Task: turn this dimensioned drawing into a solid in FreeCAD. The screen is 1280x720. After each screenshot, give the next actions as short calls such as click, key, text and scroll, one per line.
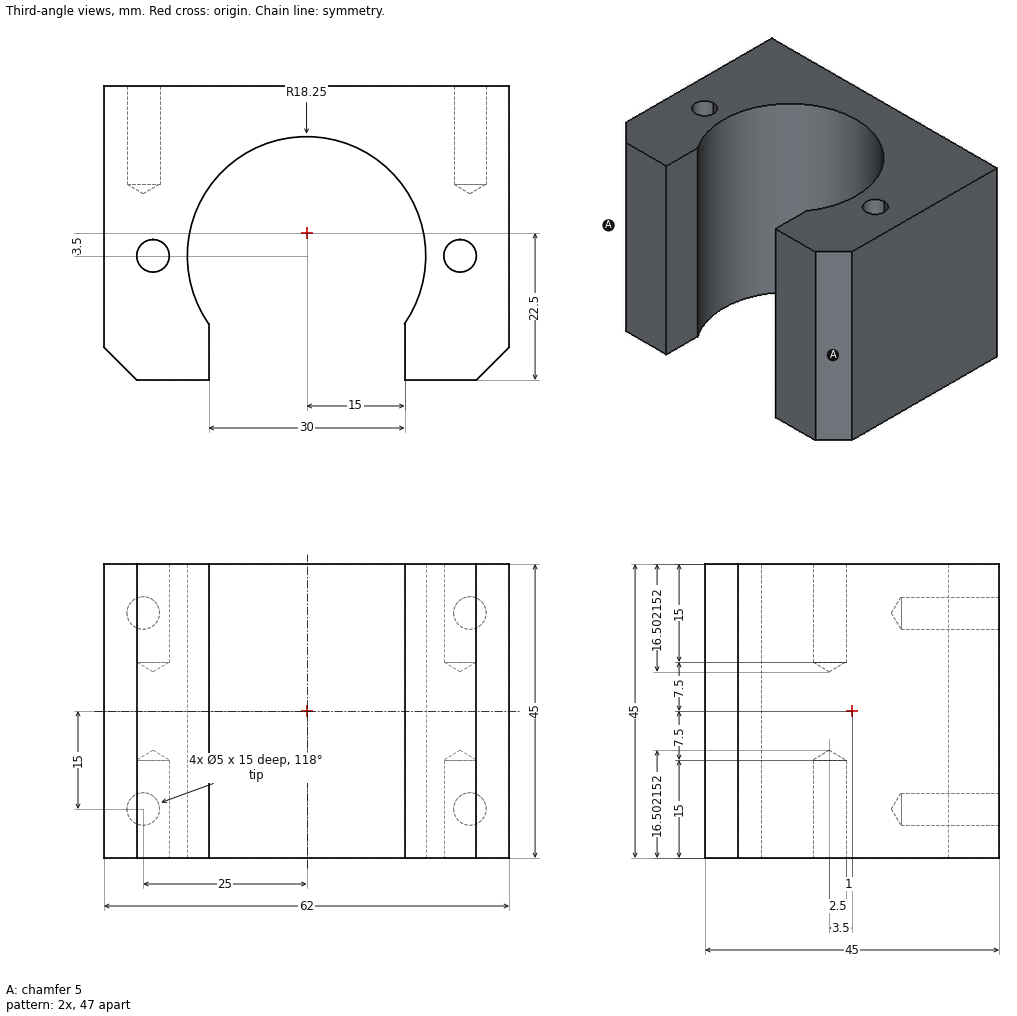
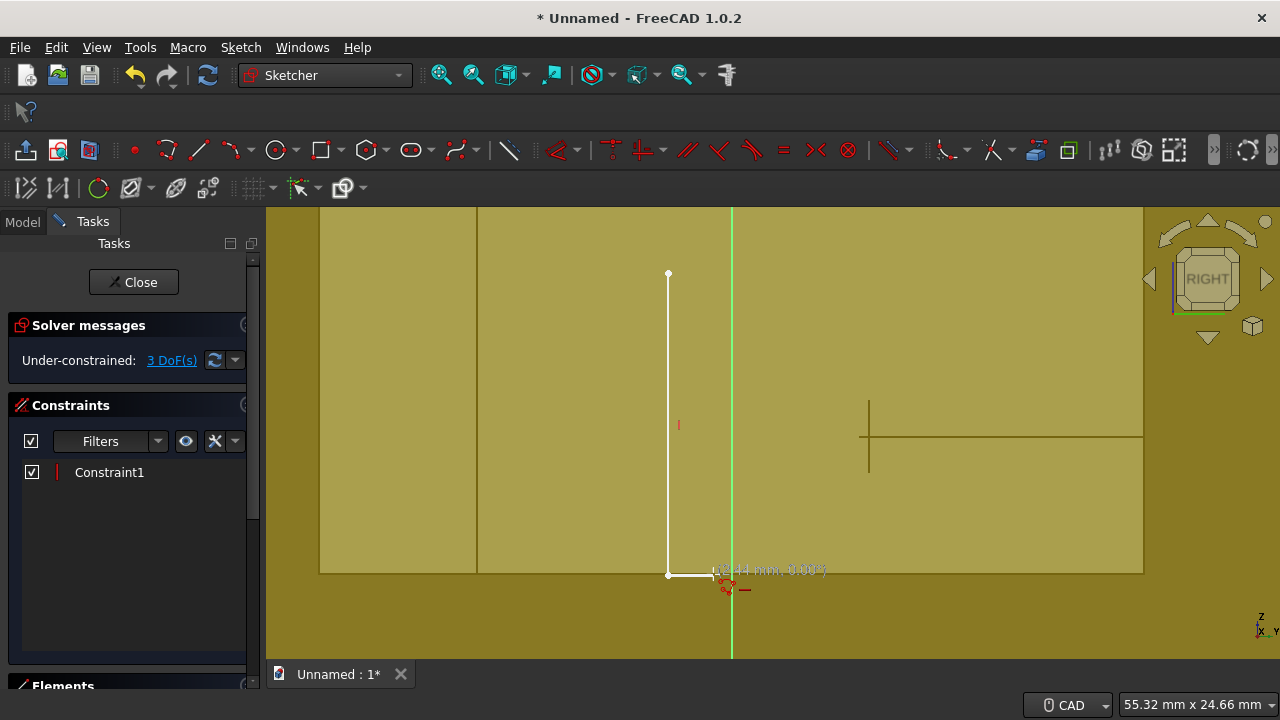
click(713, 574)
click(713, 299)
click(668, 274)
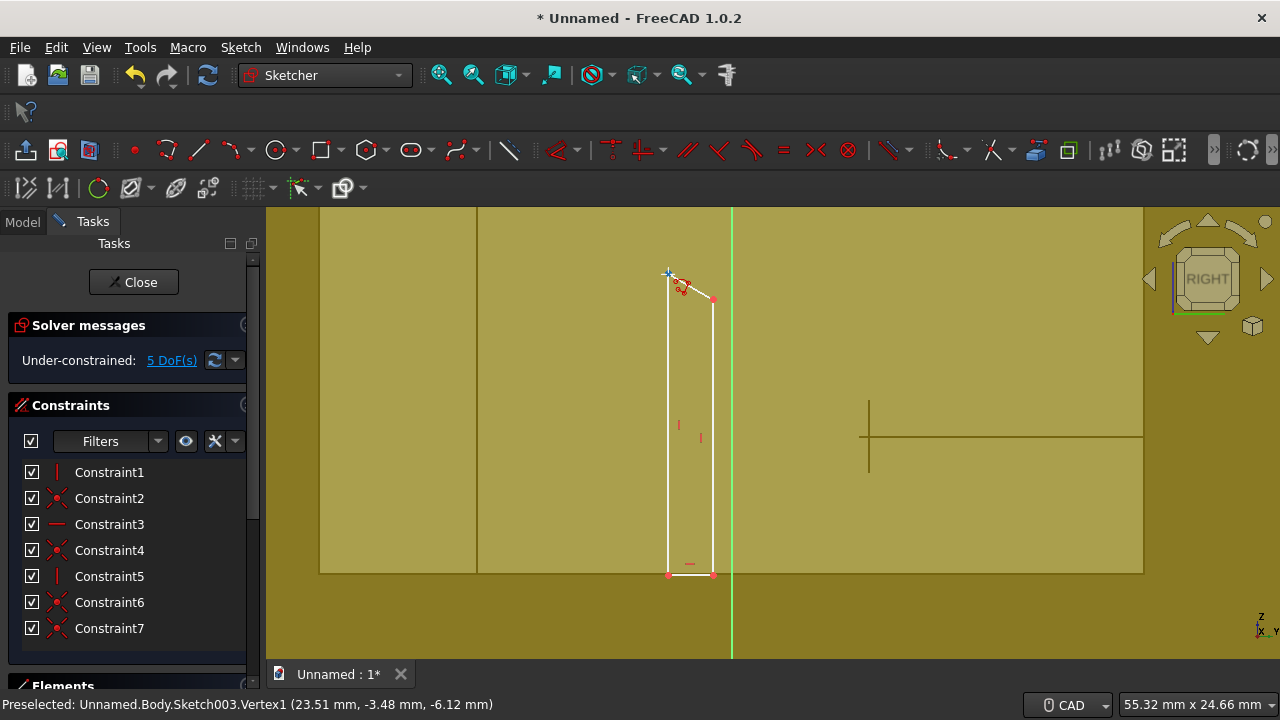
click(200, 150)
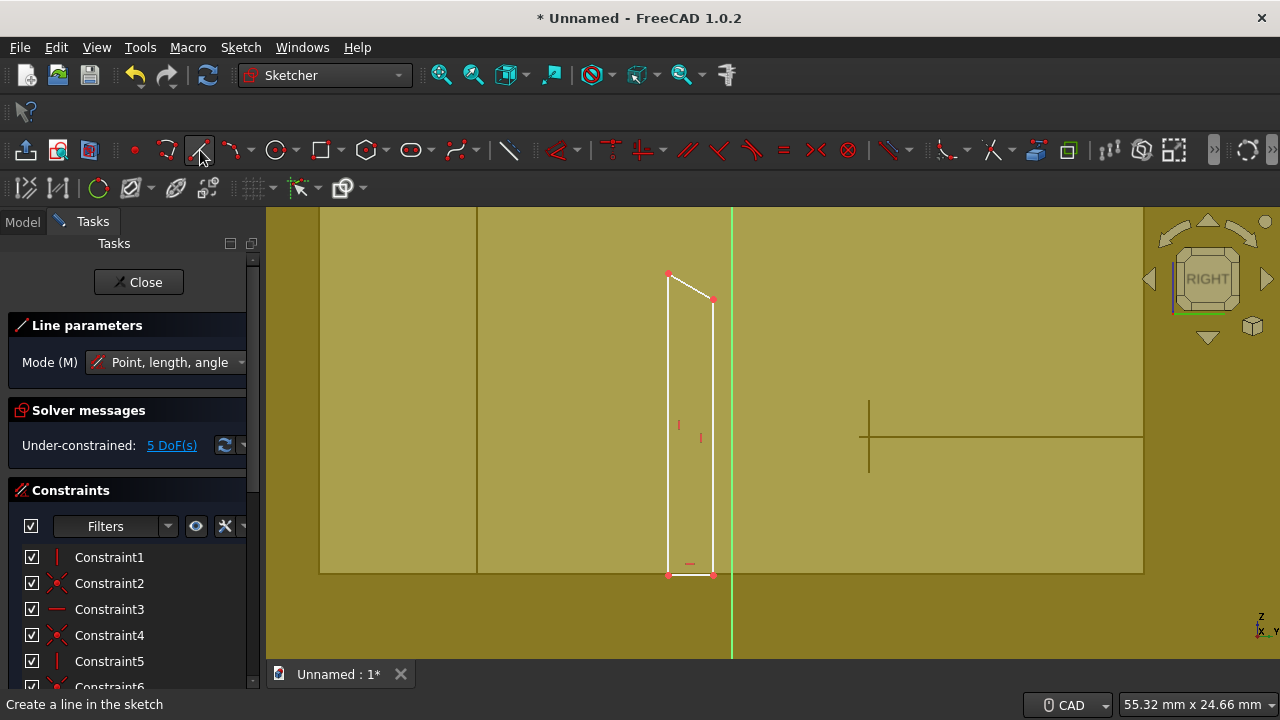
click(668, 241)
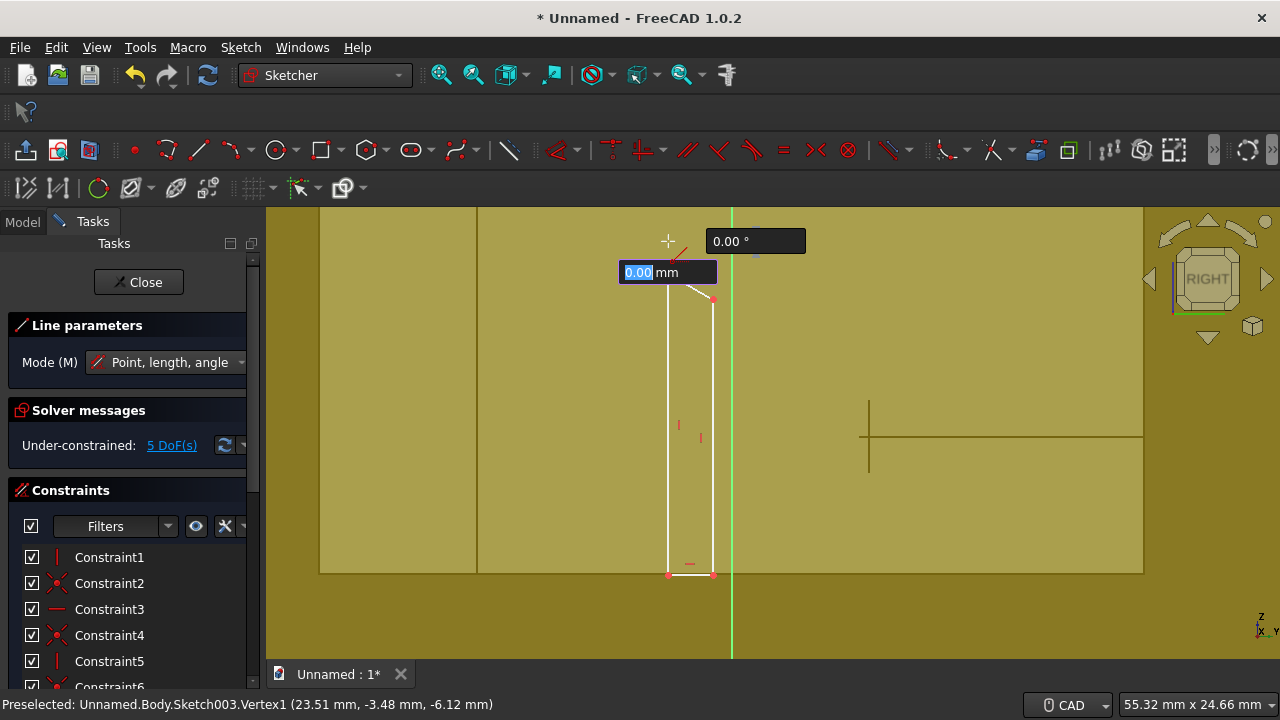
scroll(714, 577, down, 2)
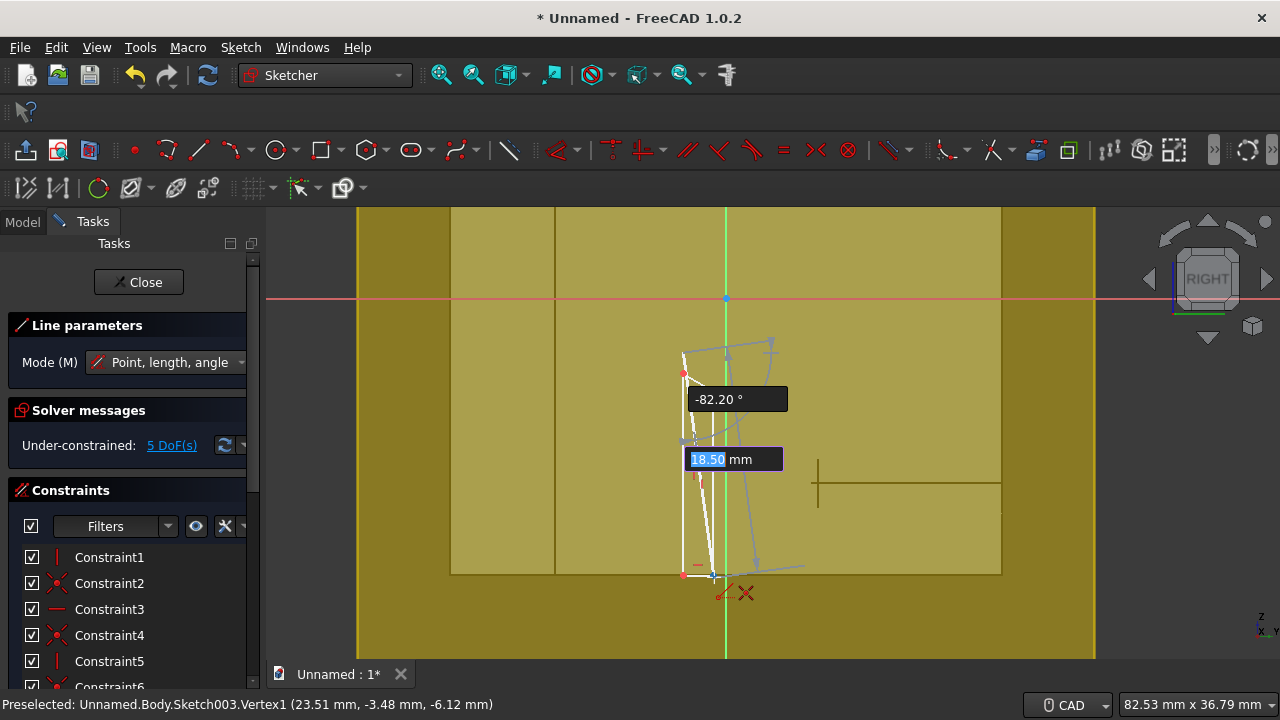
scroll(683, 291, up, 4)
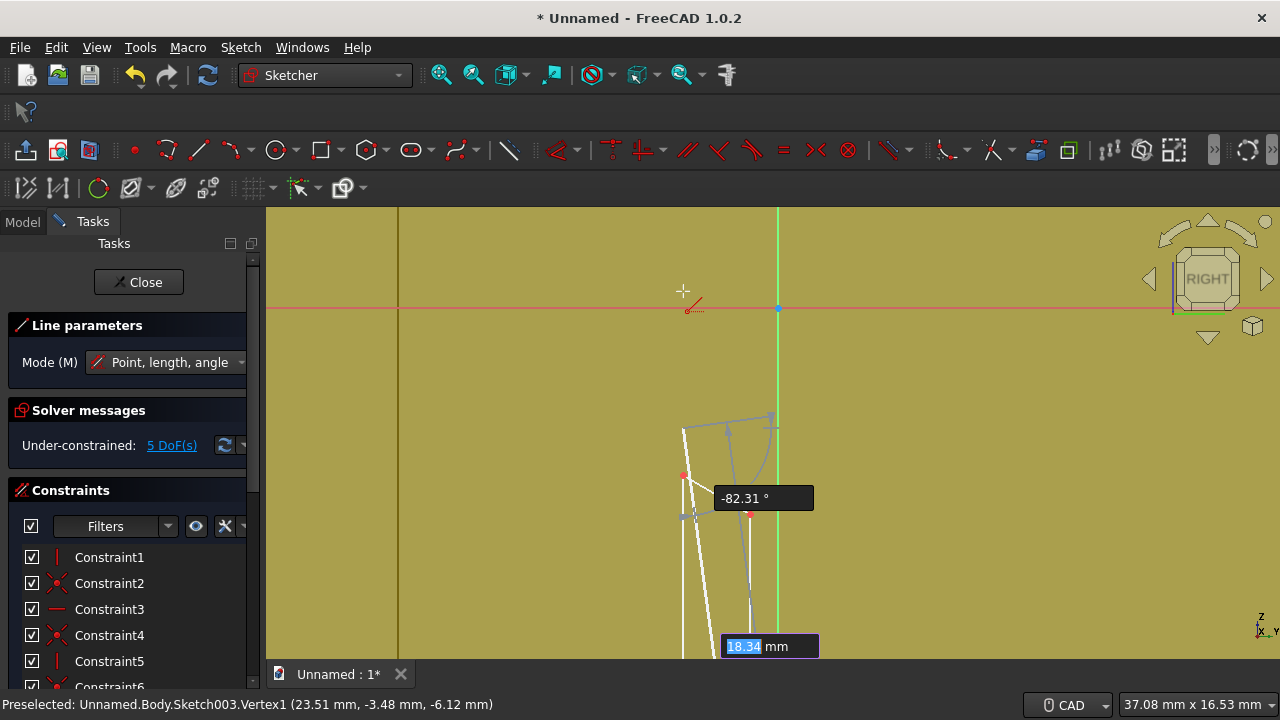
click(683, 292)
key(Escape)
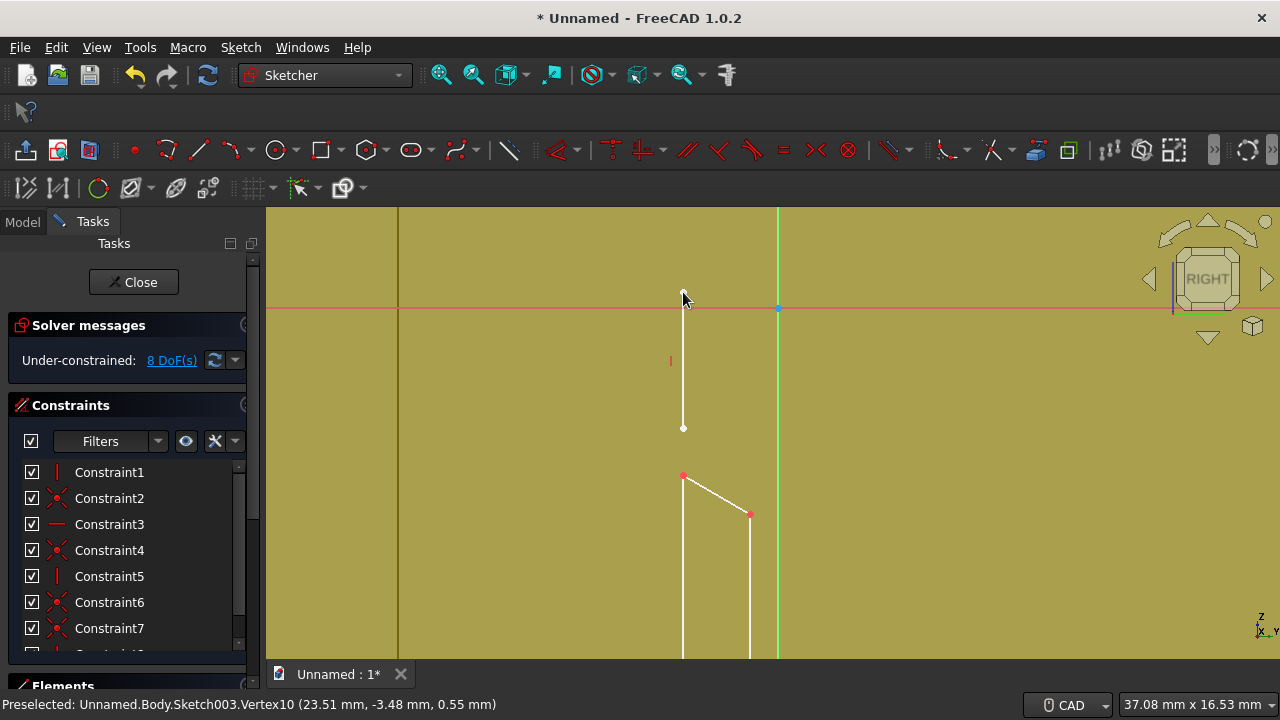
click(683, 388)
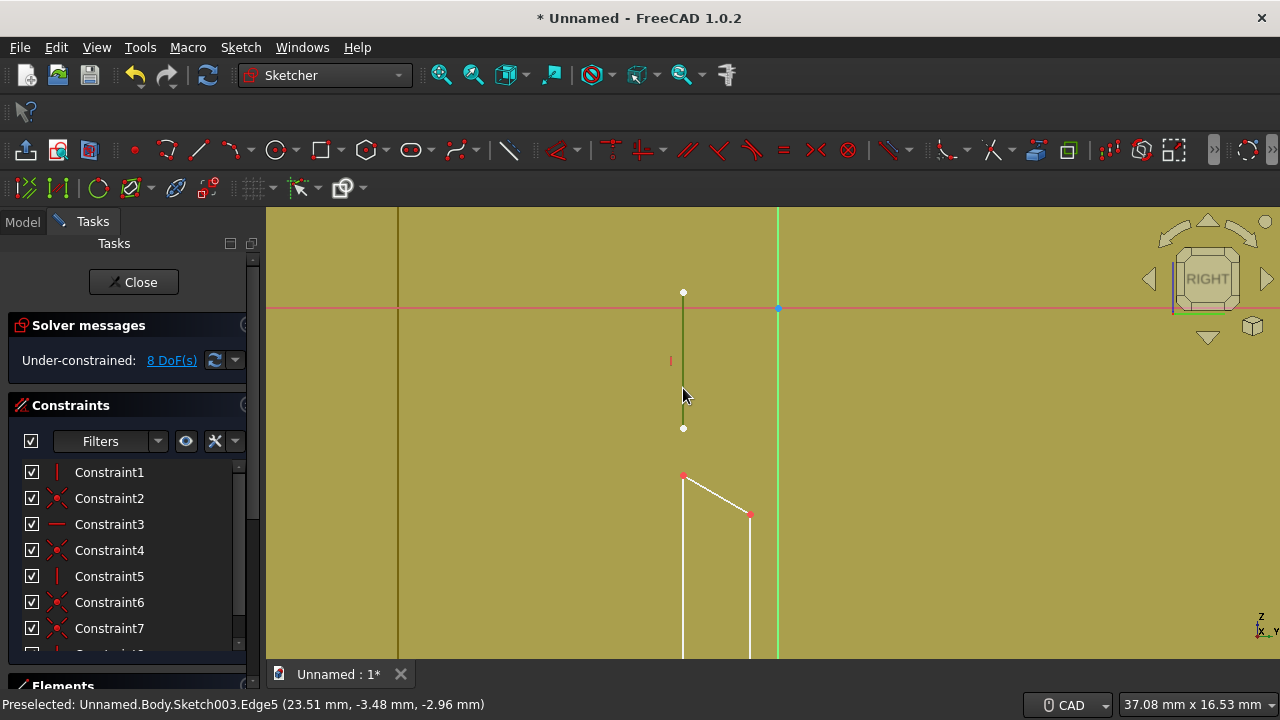
click(510, 150)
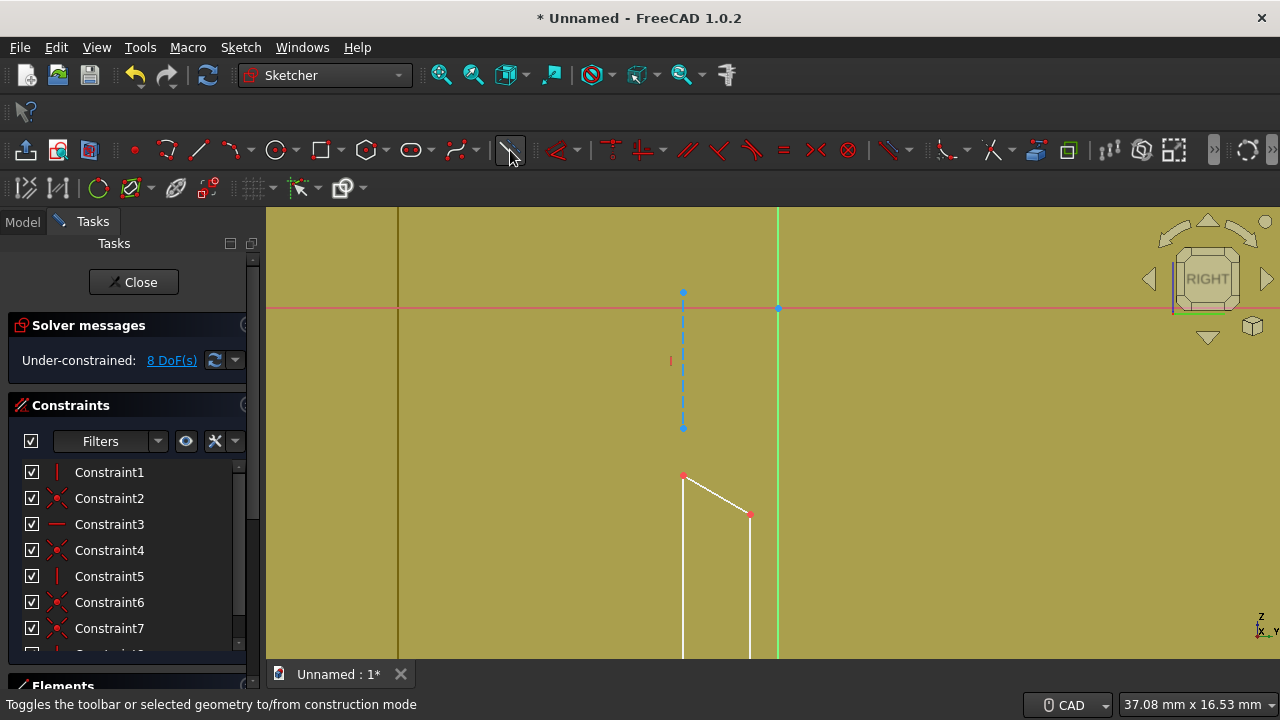
click(556, 150)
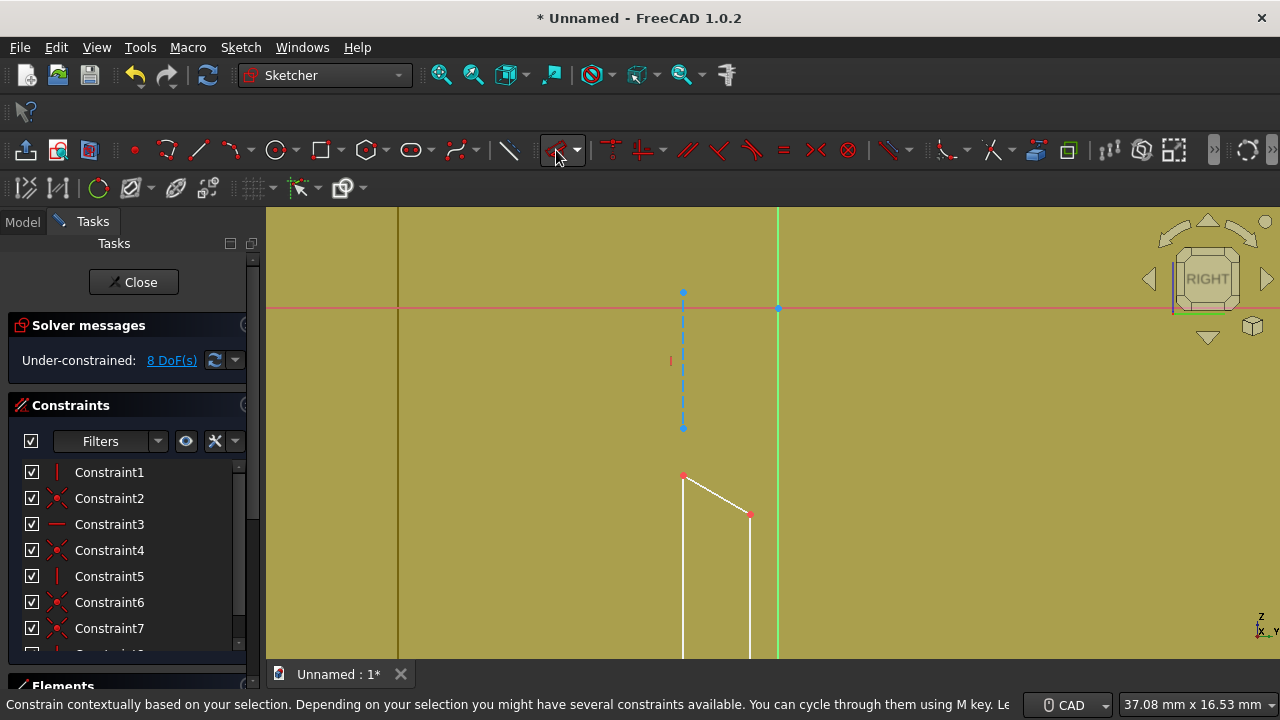
click(750, 597)
click(716, 573)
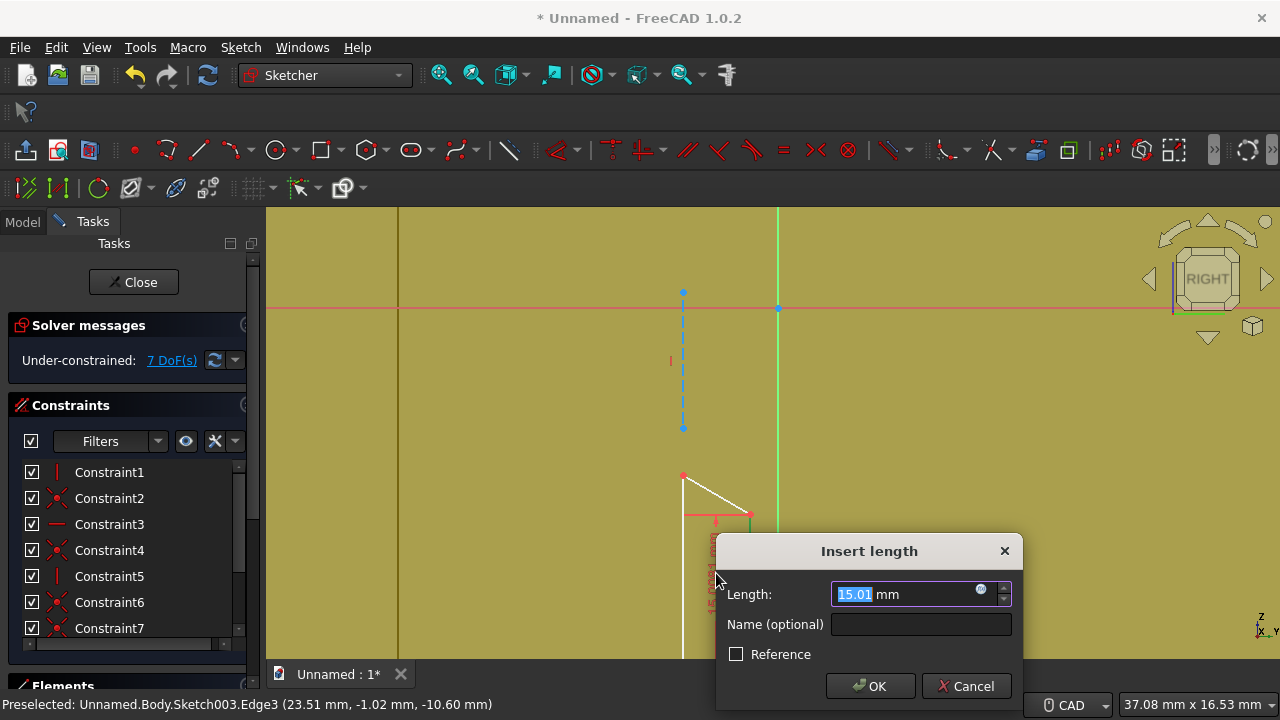
text(15)
key(Return)